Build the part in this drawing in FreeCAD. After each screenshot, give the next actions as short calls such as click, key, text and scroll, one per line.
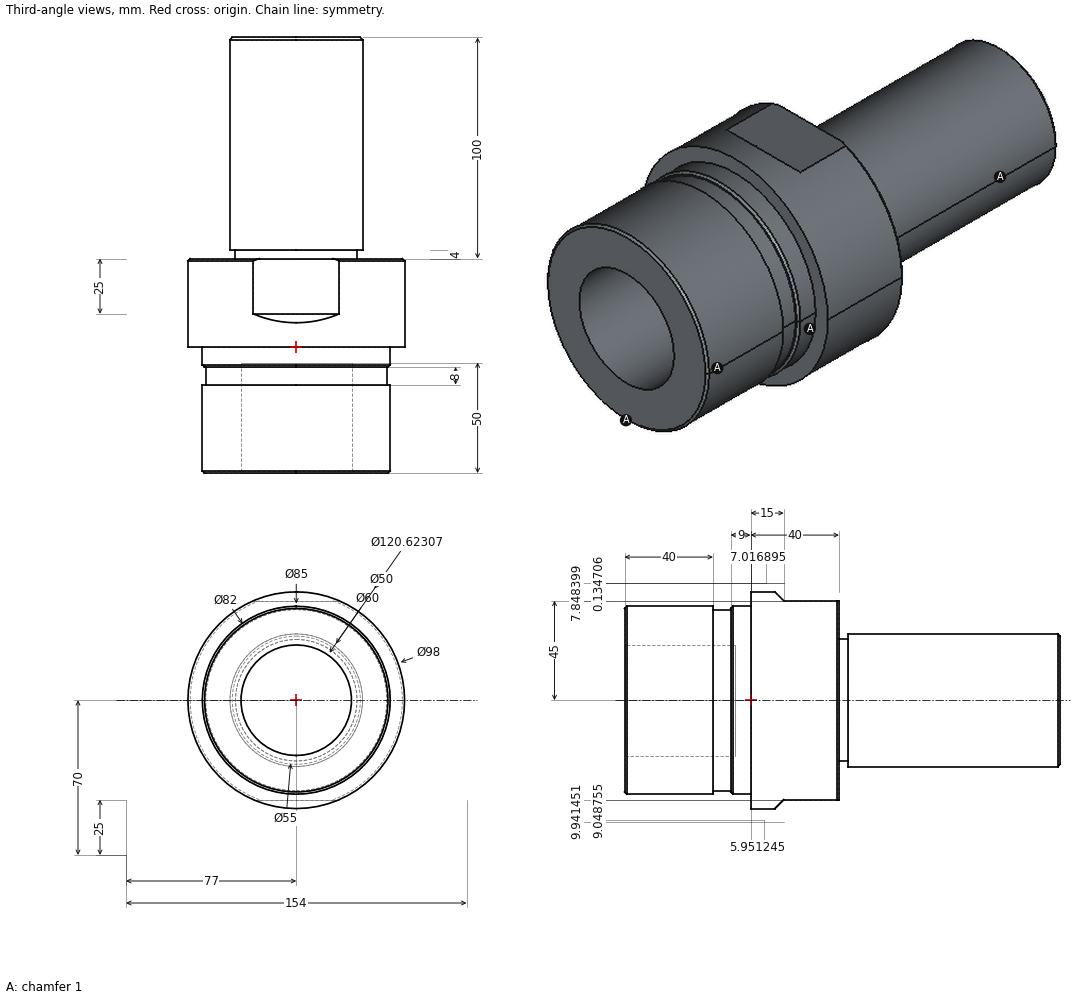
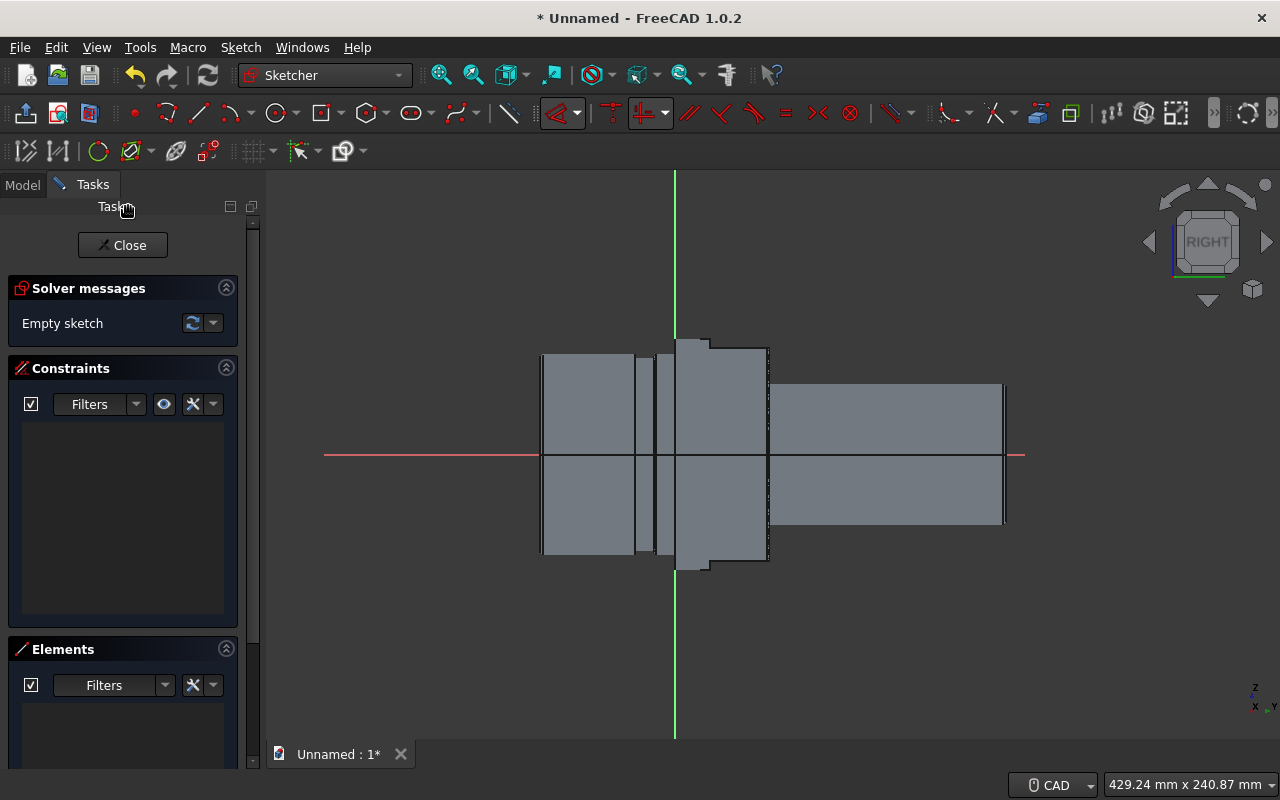
click(90, 114)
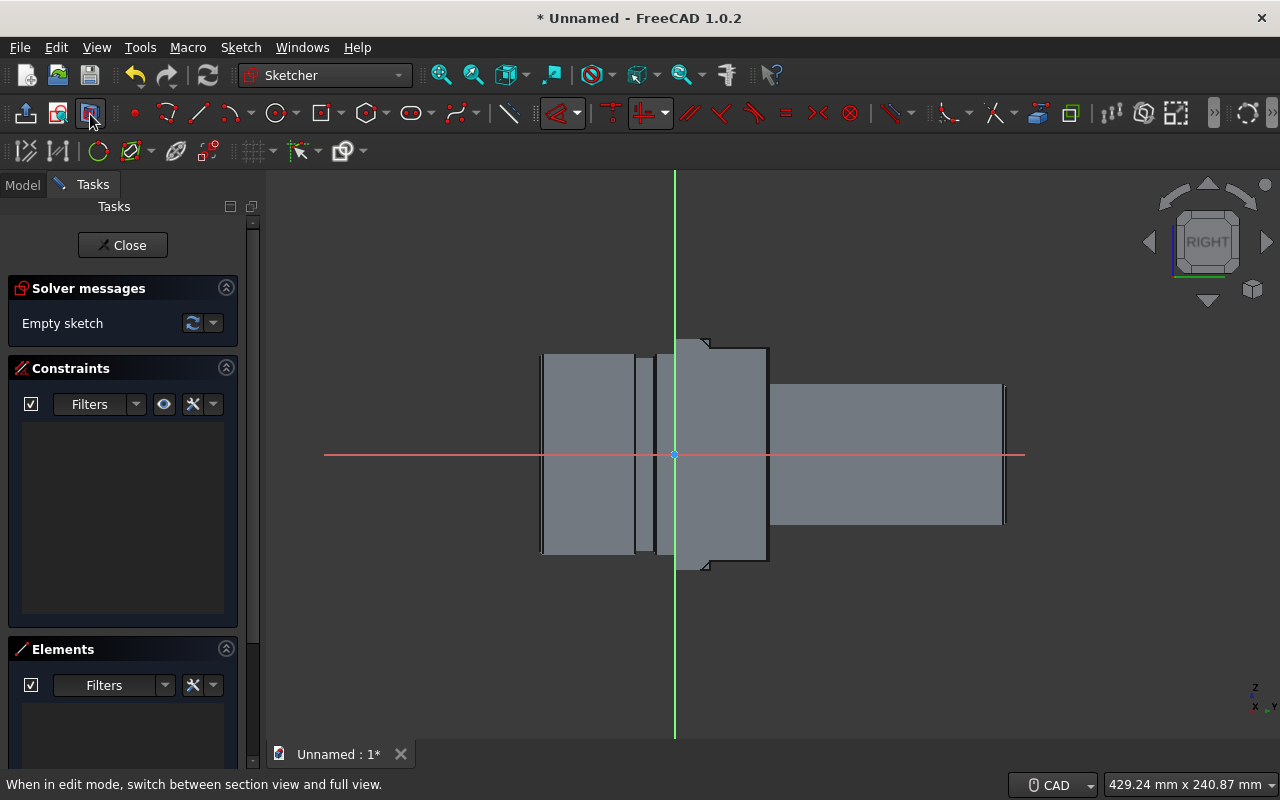
scroll(669, 462, up, 2)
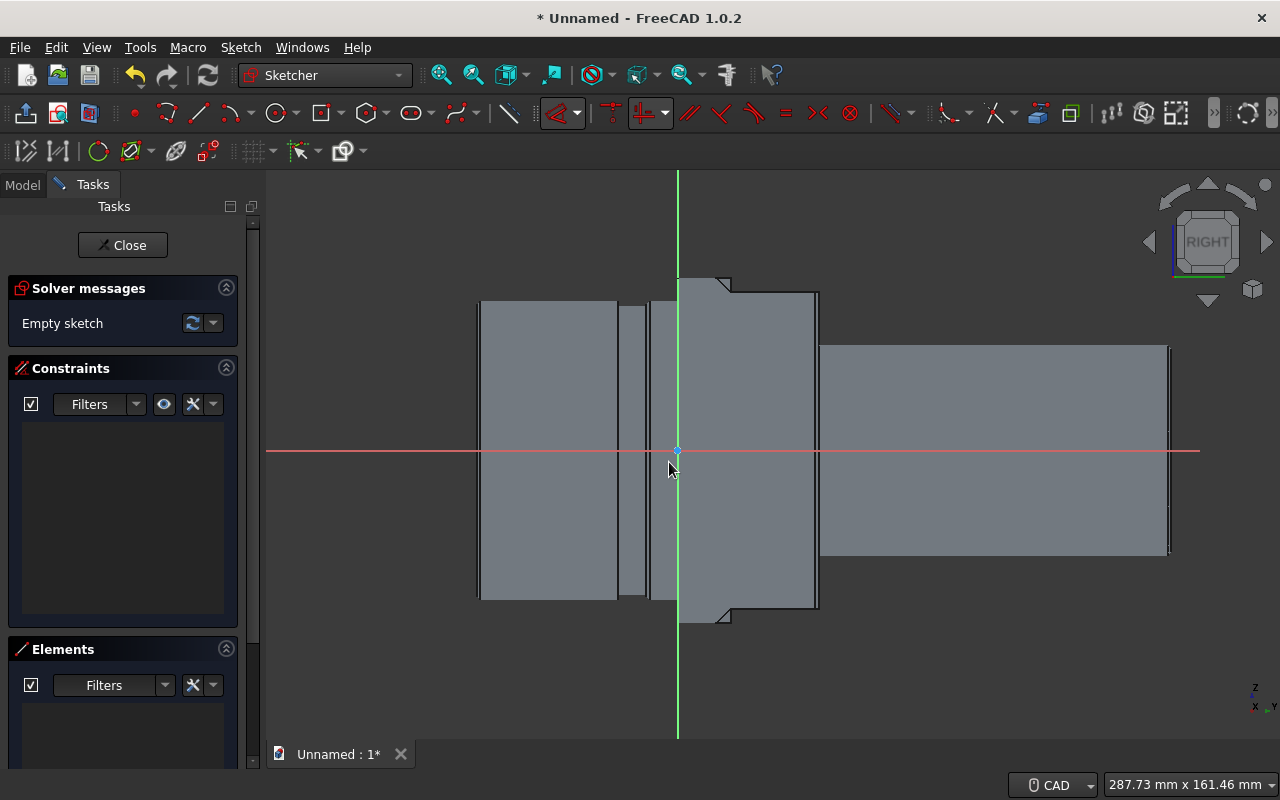
click(168, 114)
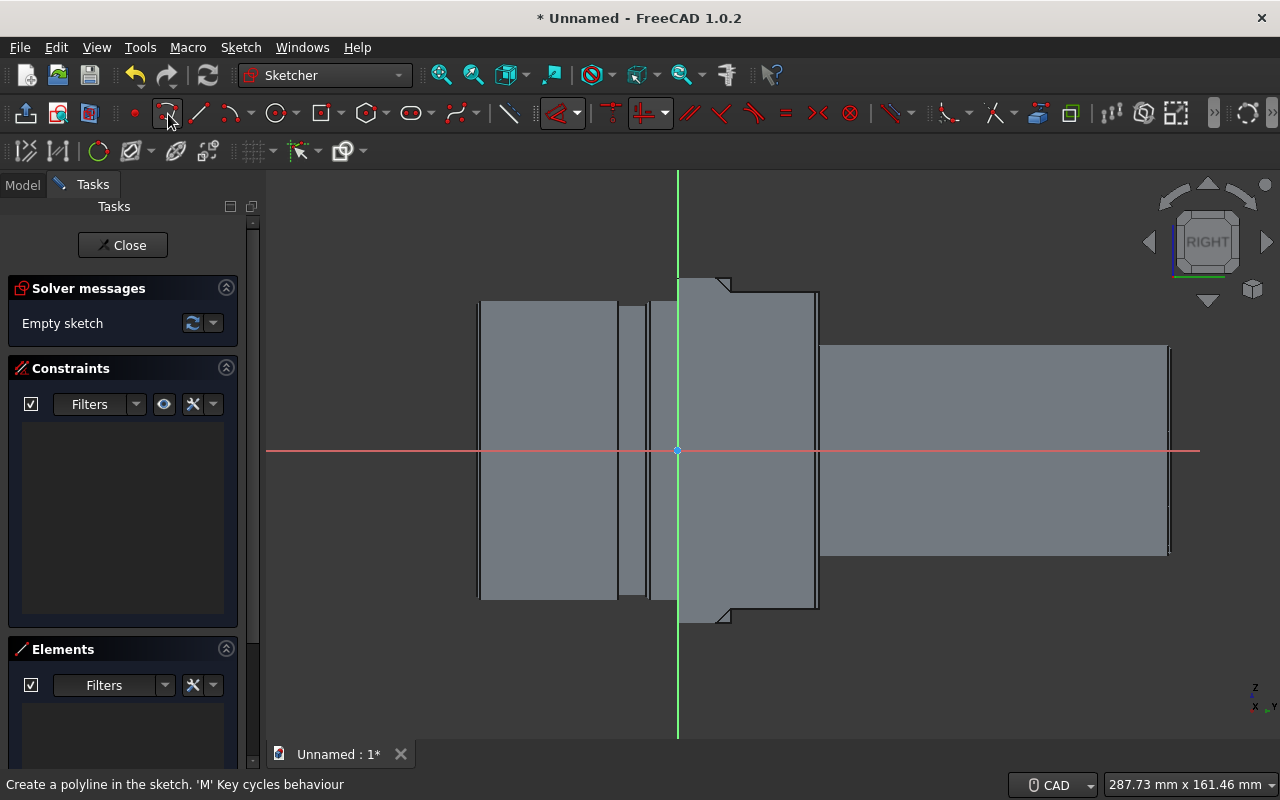
click(731, 292)
click(731, 264)
click(702, 261)
click(731, 293)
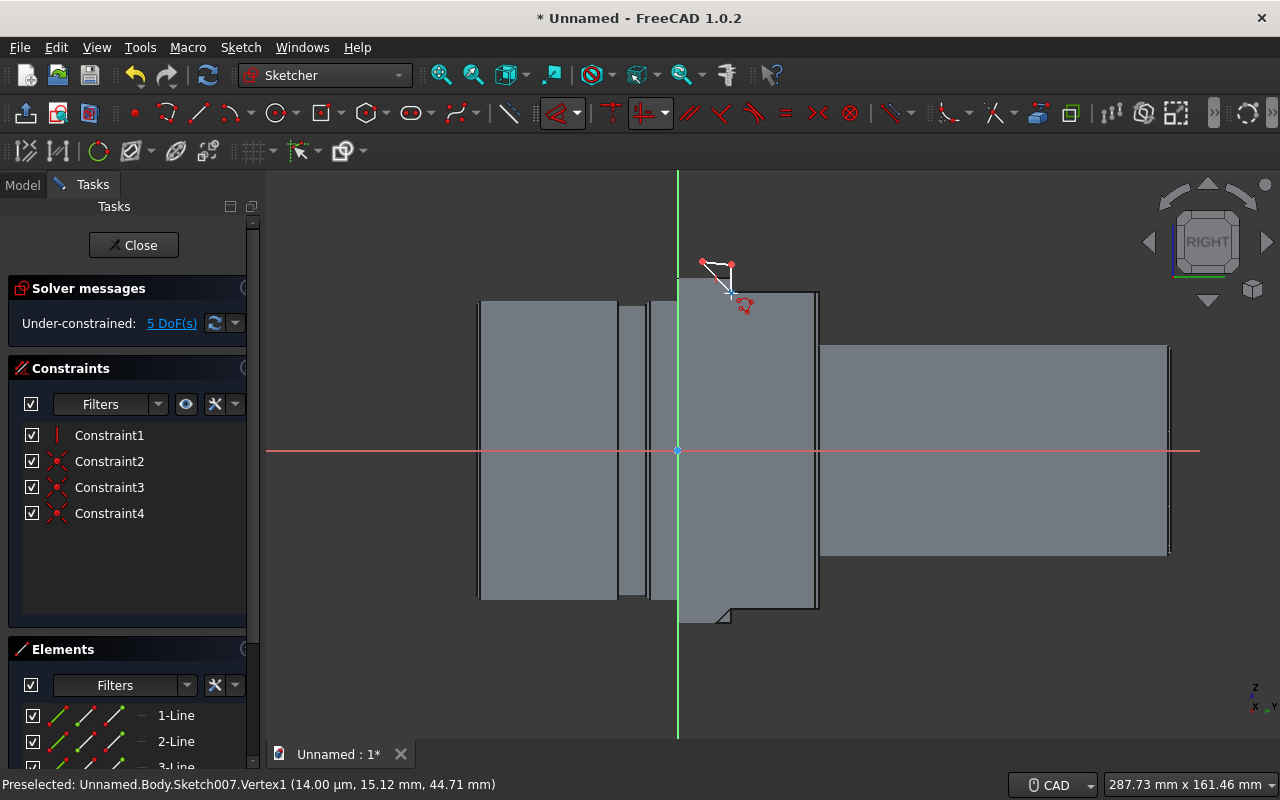
click(731, 609)
click(699, 641)
click(731, 644)
click(731, 610)
key(Escape)
key(Escape)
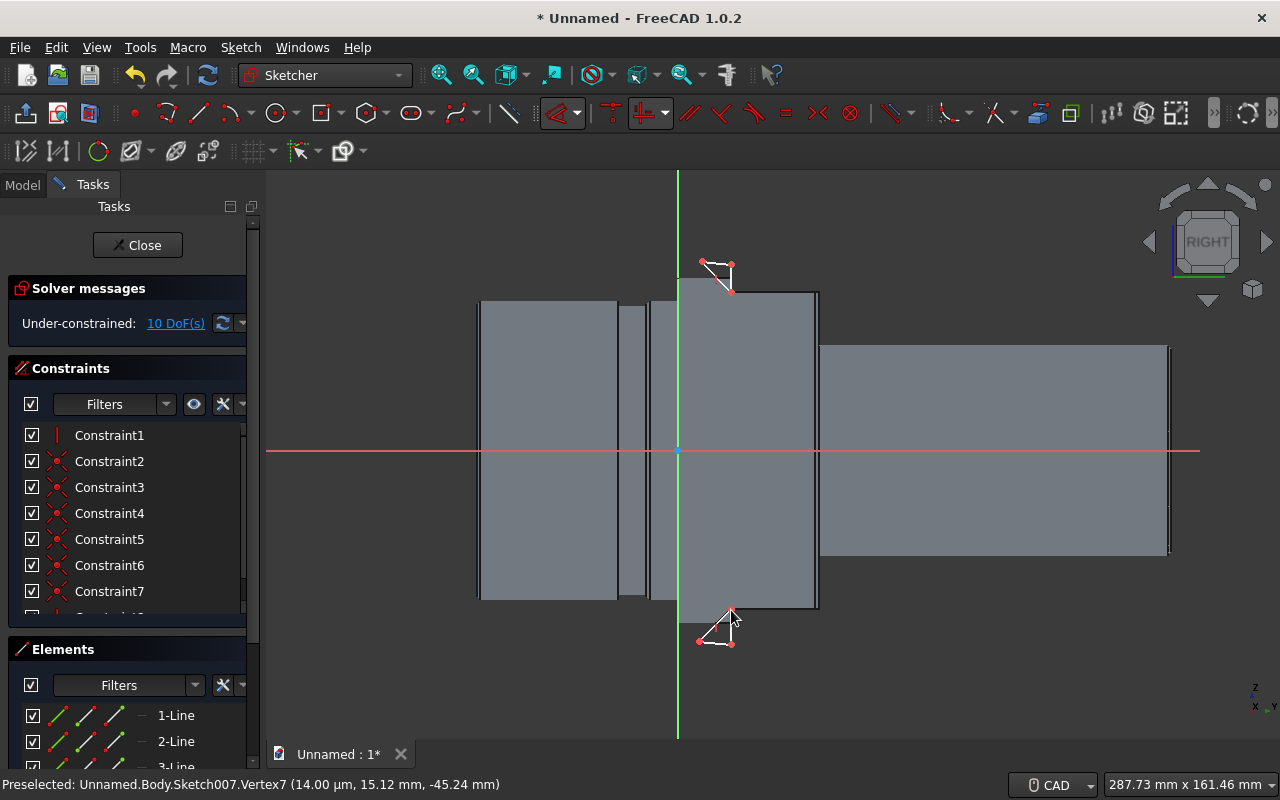
click(731, 293)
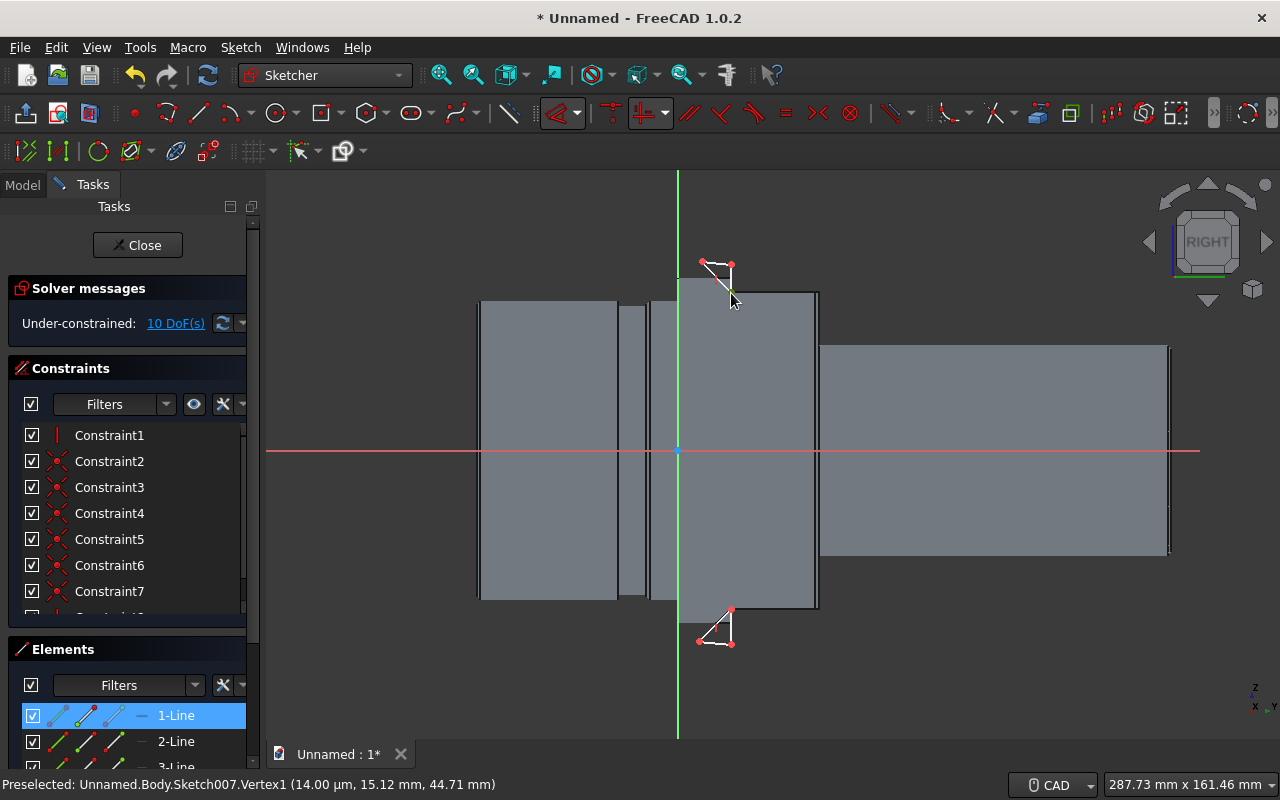
click(731, 610)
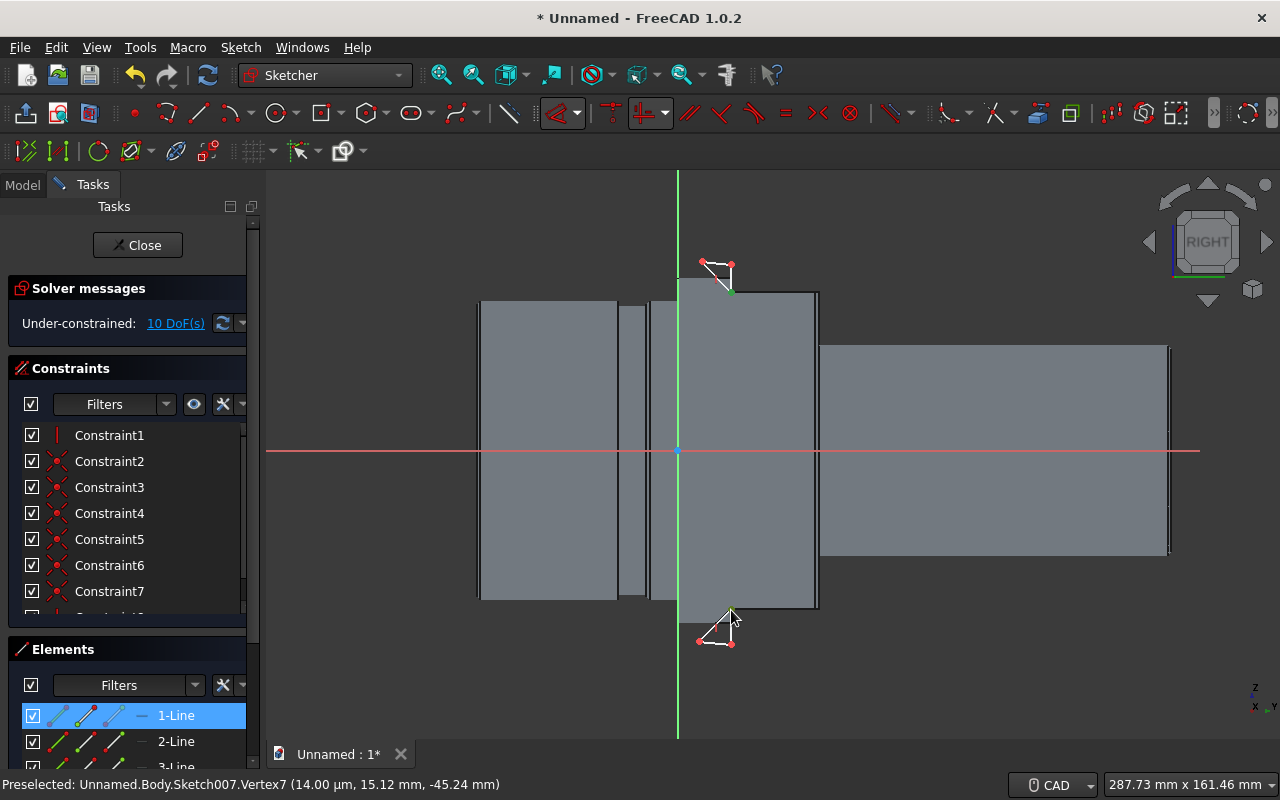
click(353, 451)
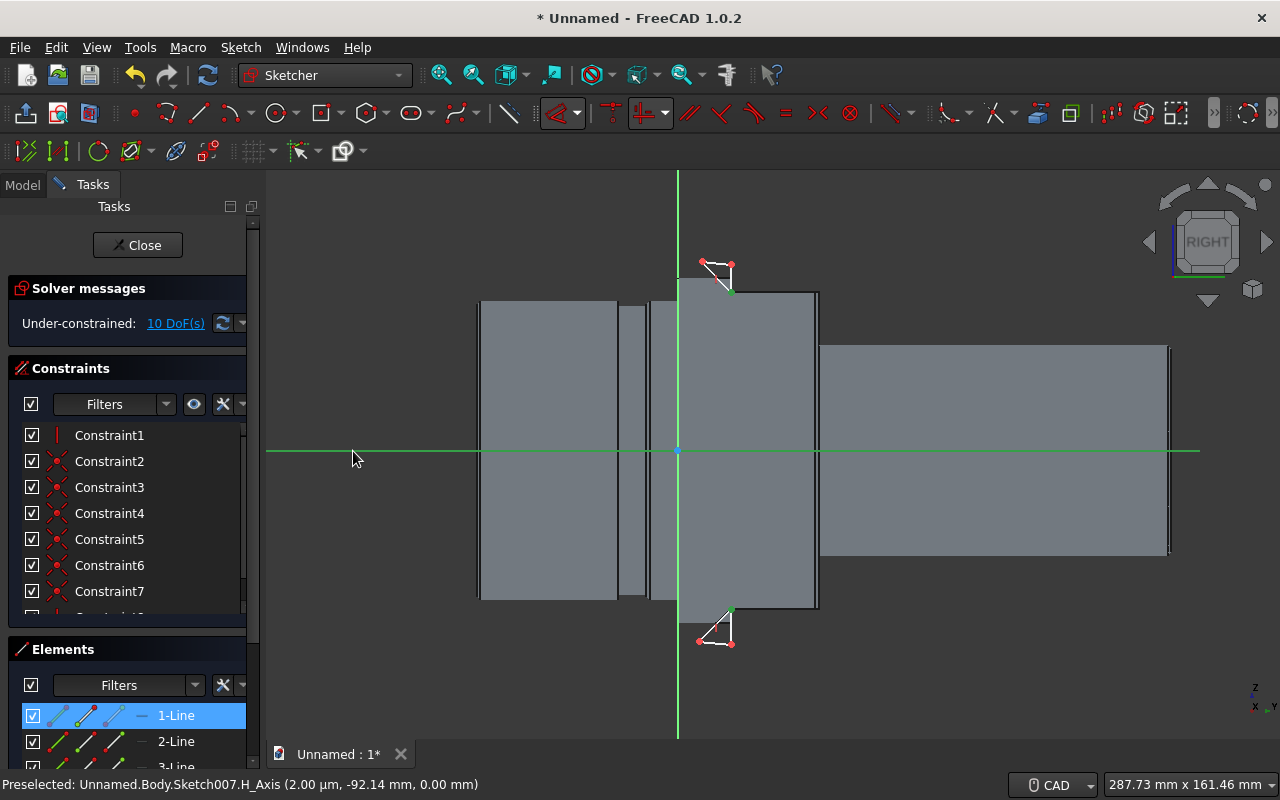
click(818, 114)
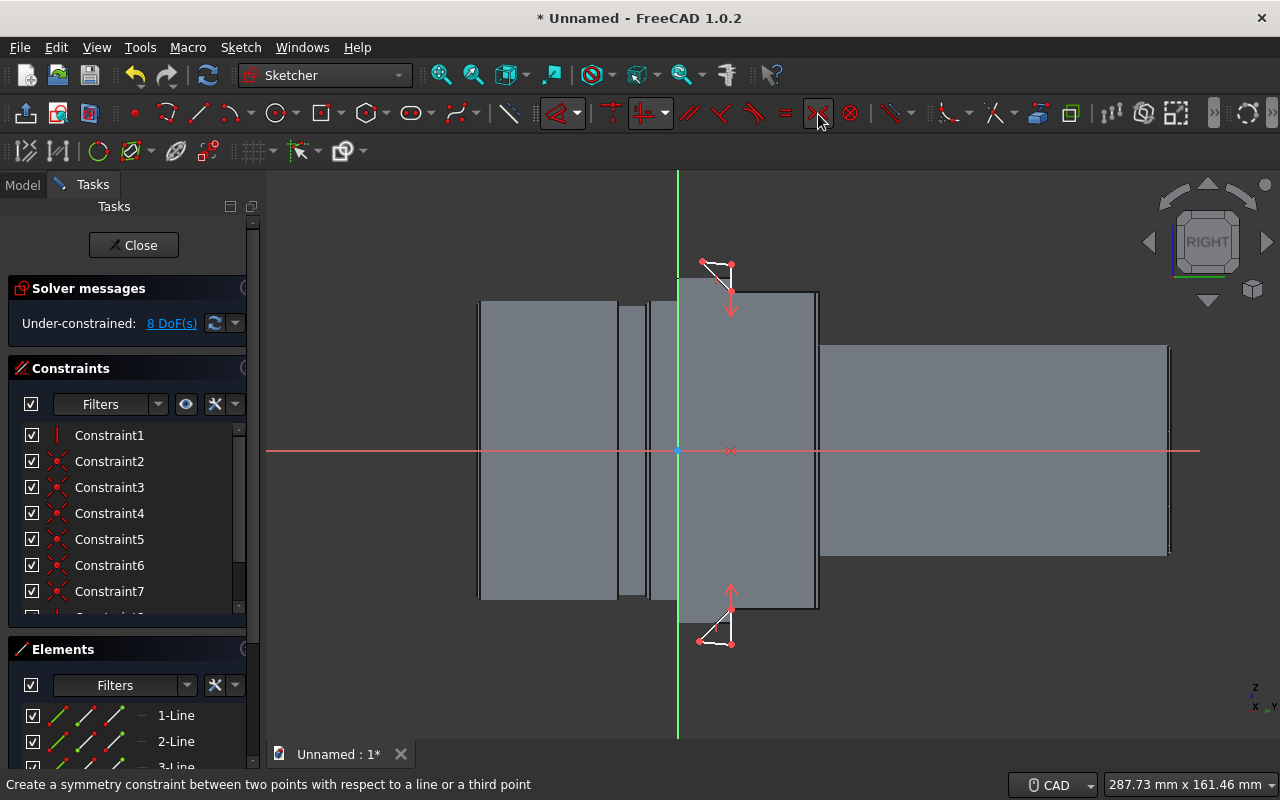
click(731, 292)